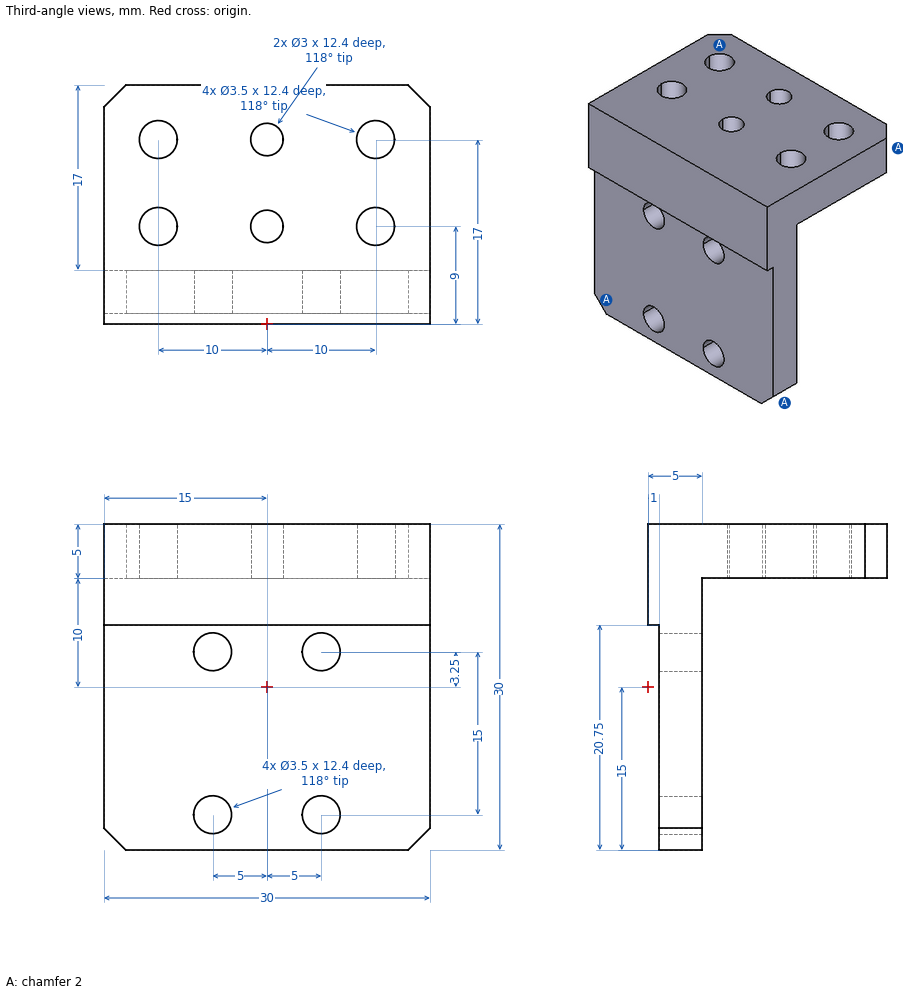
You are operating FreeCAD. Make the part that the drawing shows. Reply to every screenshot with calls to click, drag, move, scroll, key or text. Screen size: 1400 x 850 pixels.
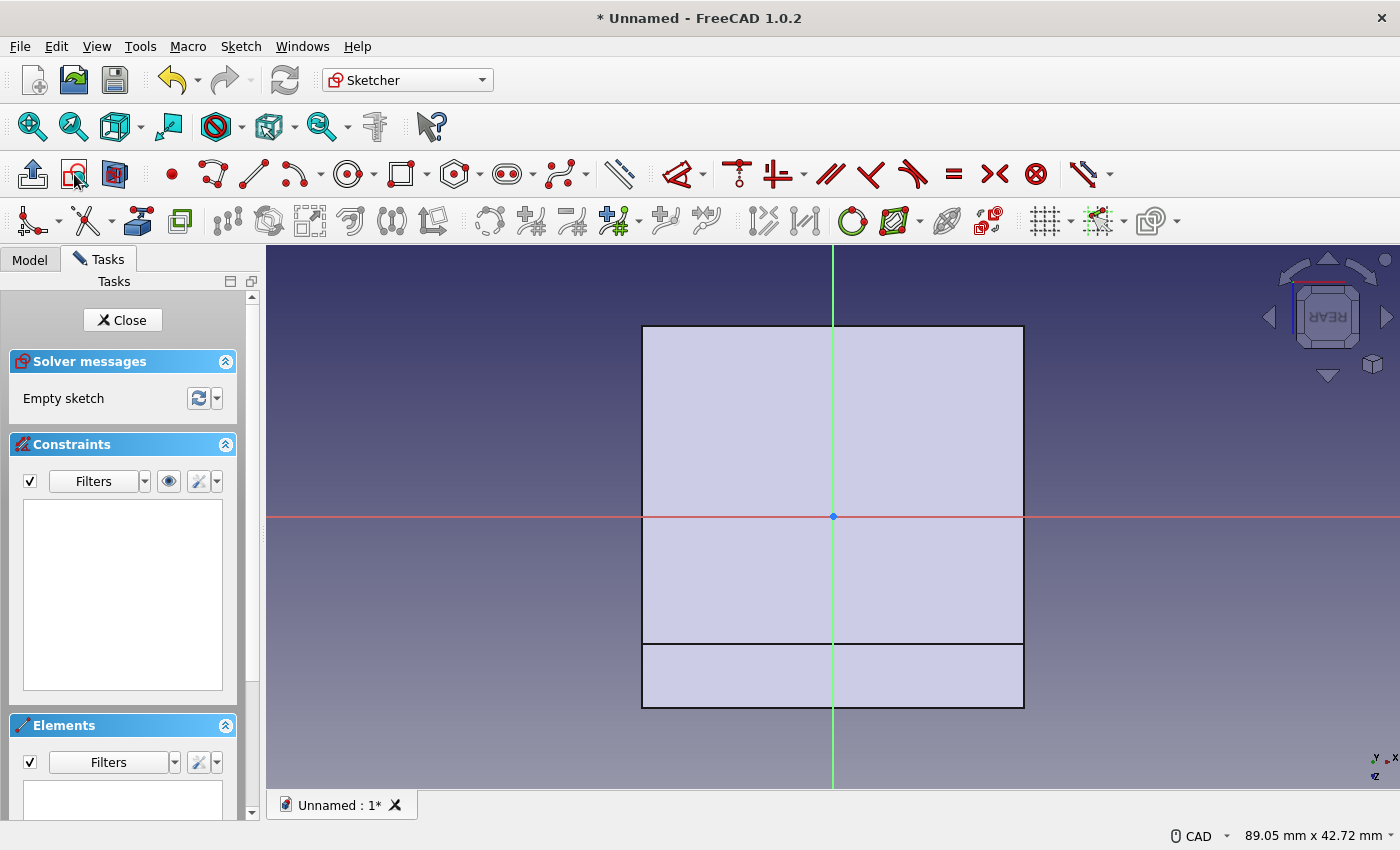
scroll(972, 353, up, 2)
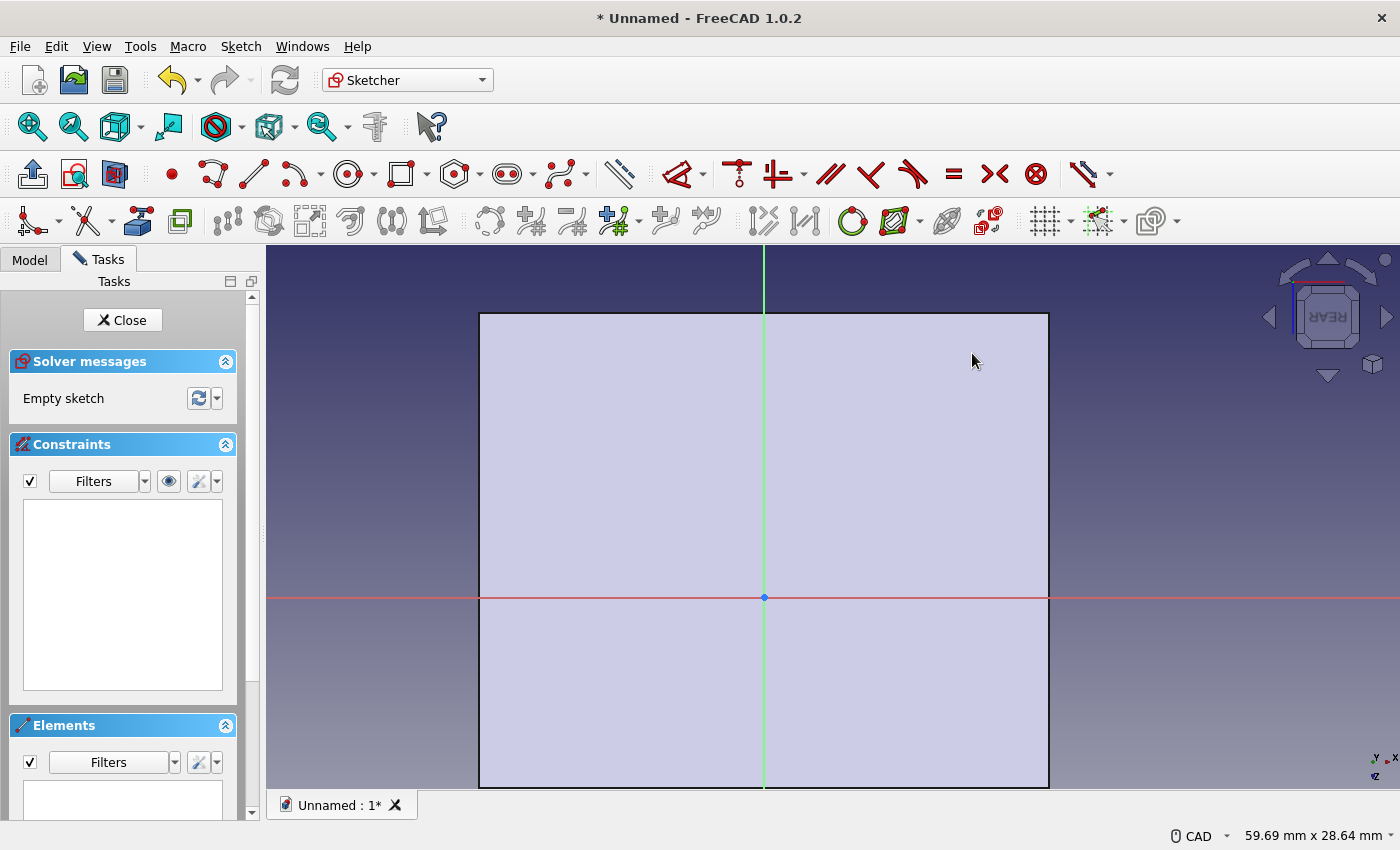
click(348, 174)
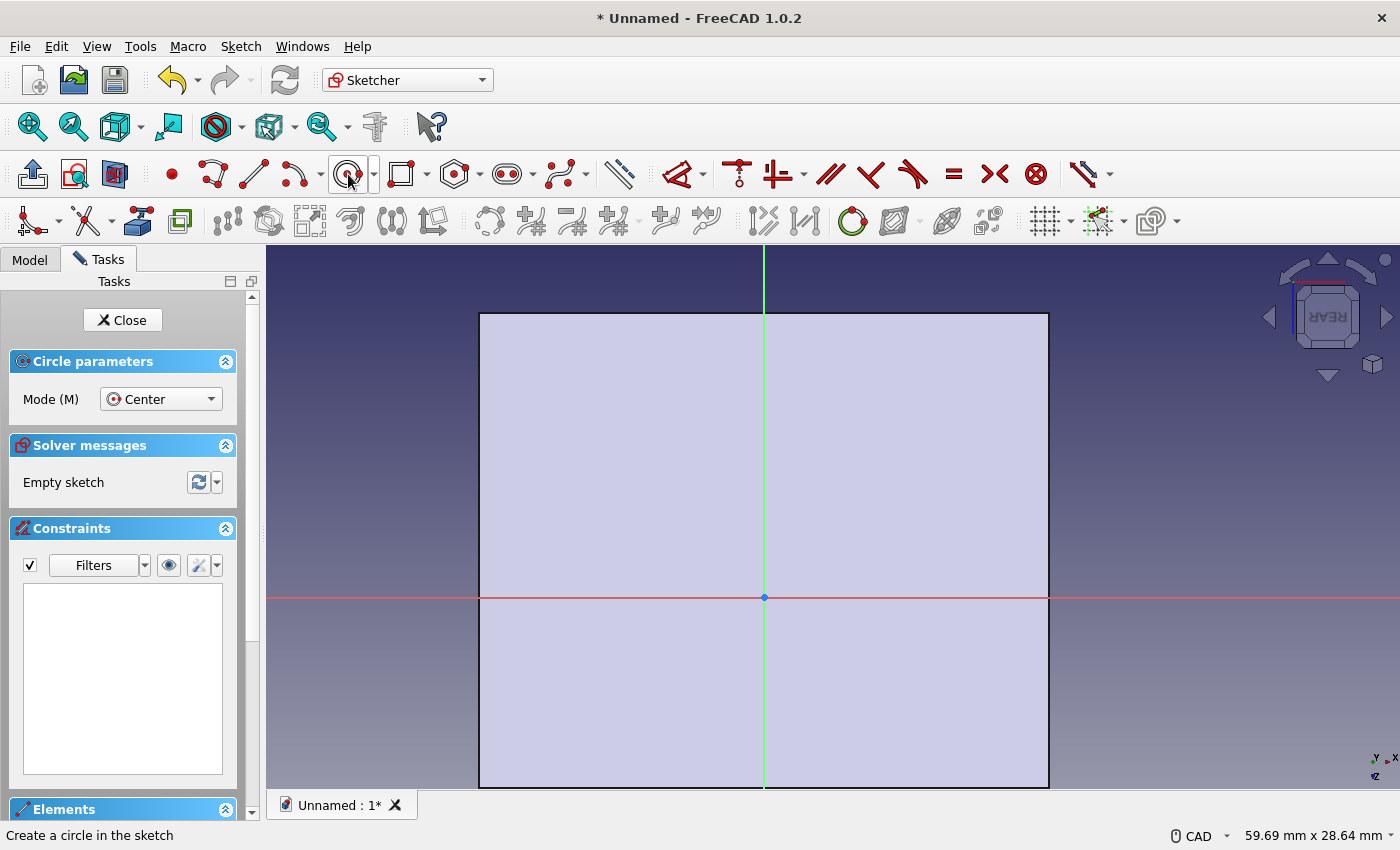
click(669, 374)
click(693, 351)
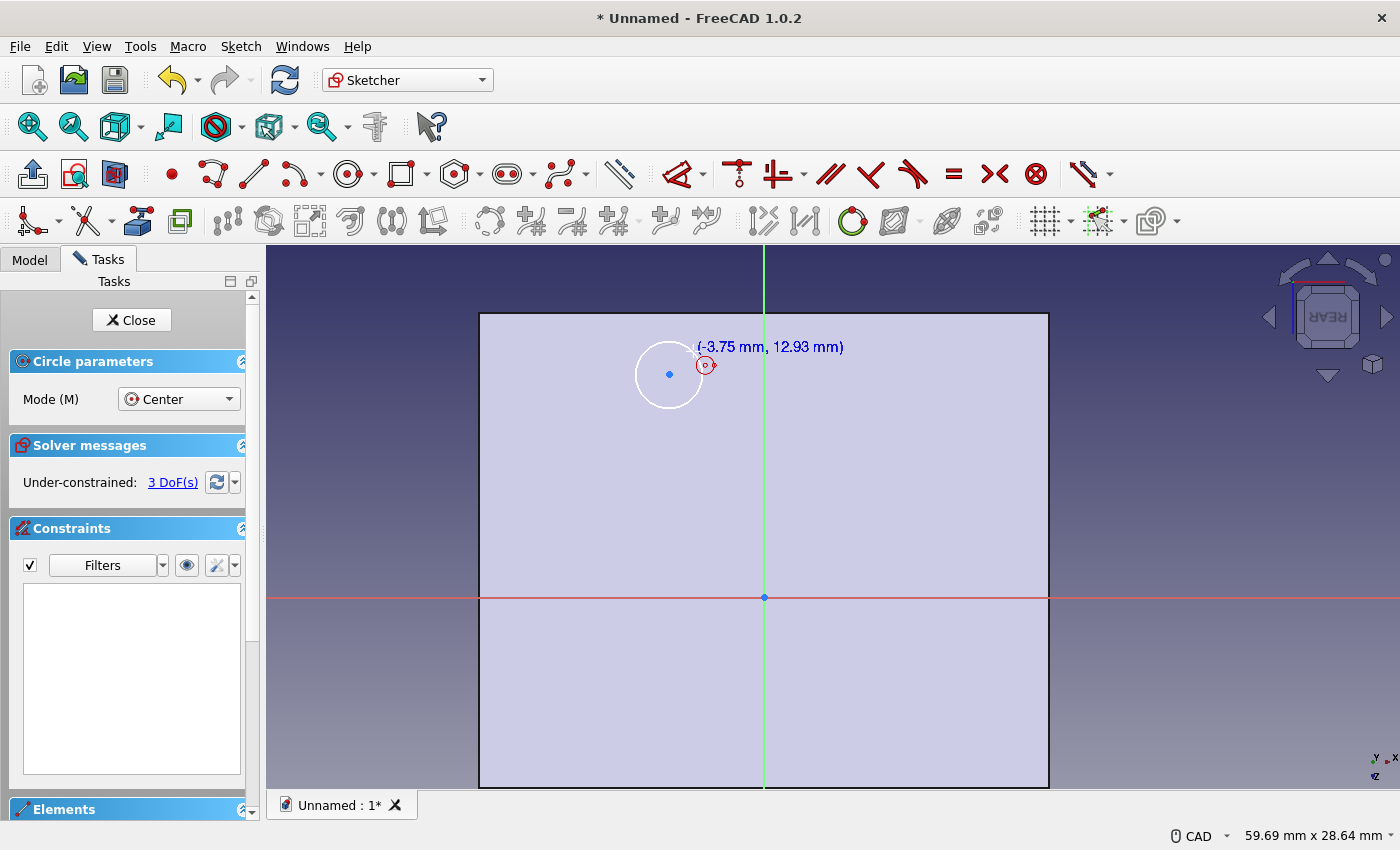
click(859, 374)
click(883, 351)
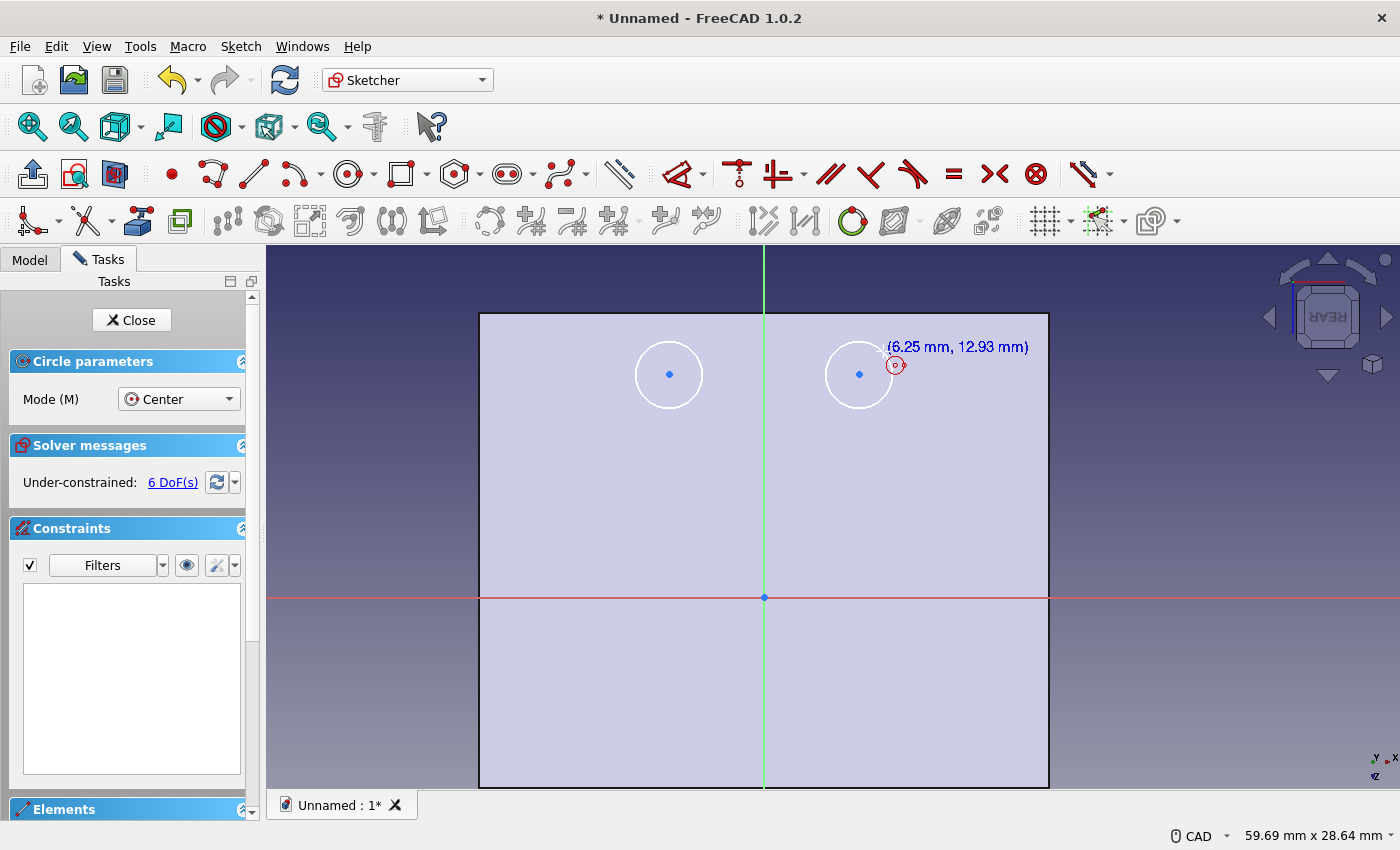
click(859, 659)
click(883, 636)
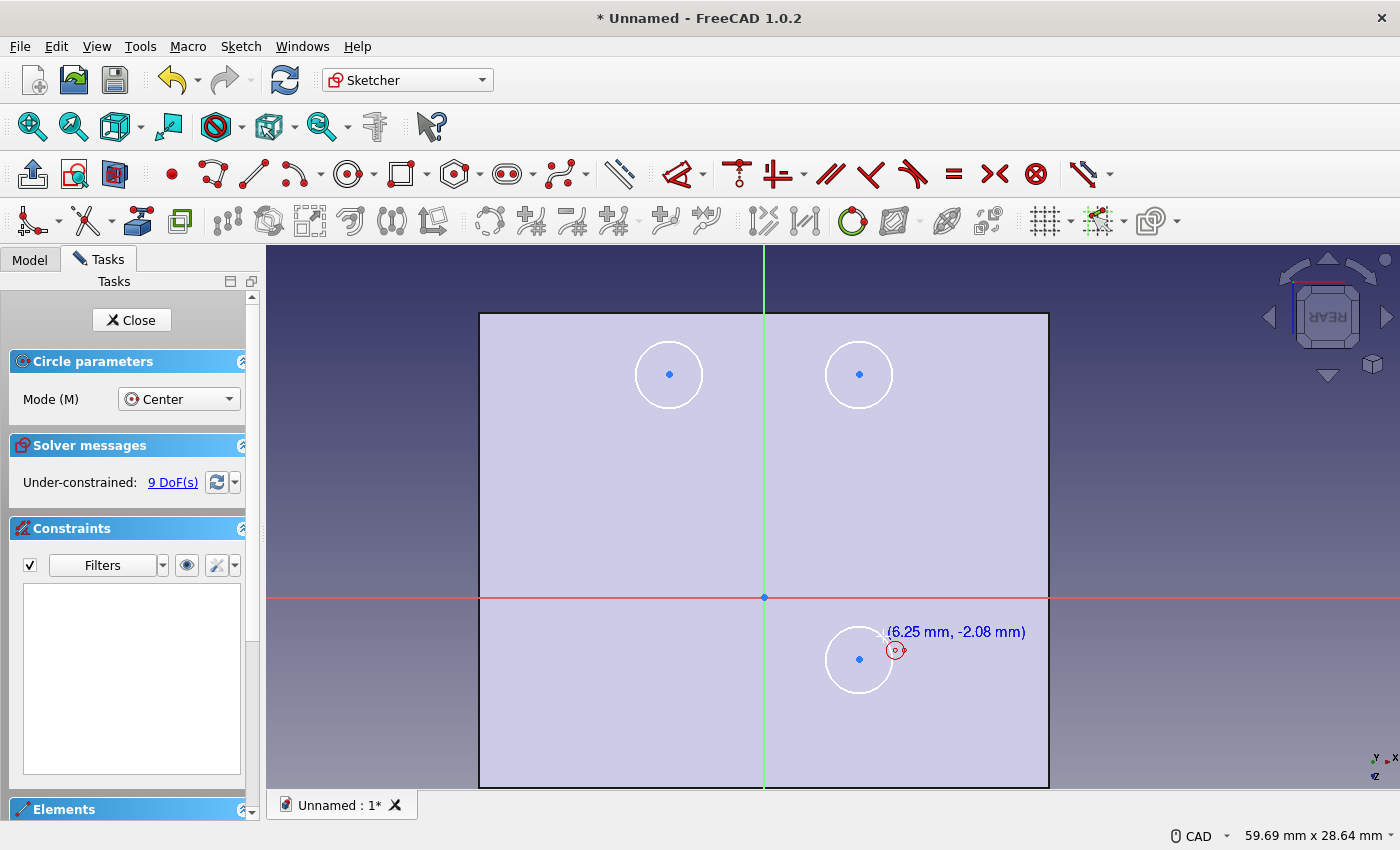
click(669, 659)
click(693, 636)
key(Escape)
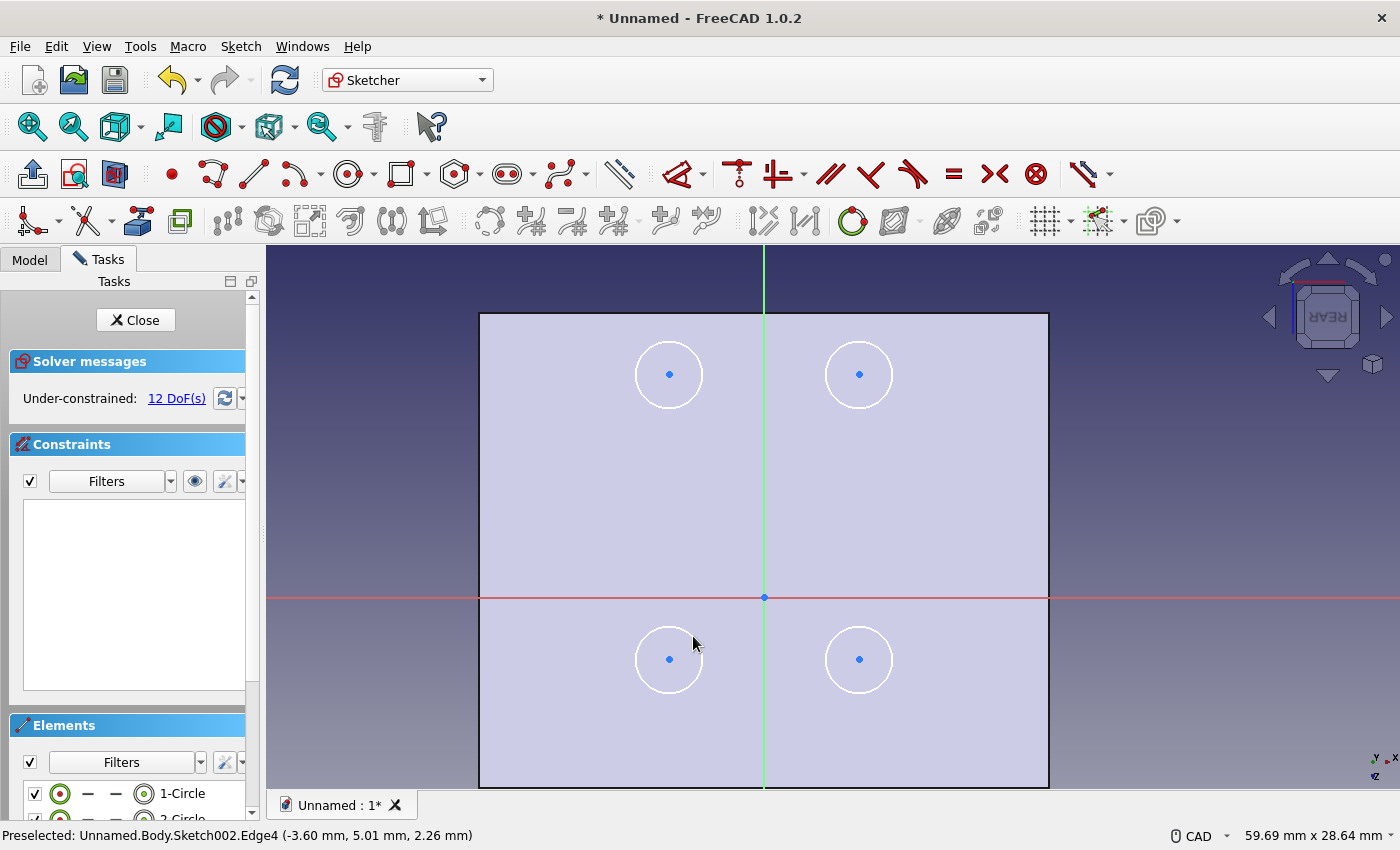
click(692, 351)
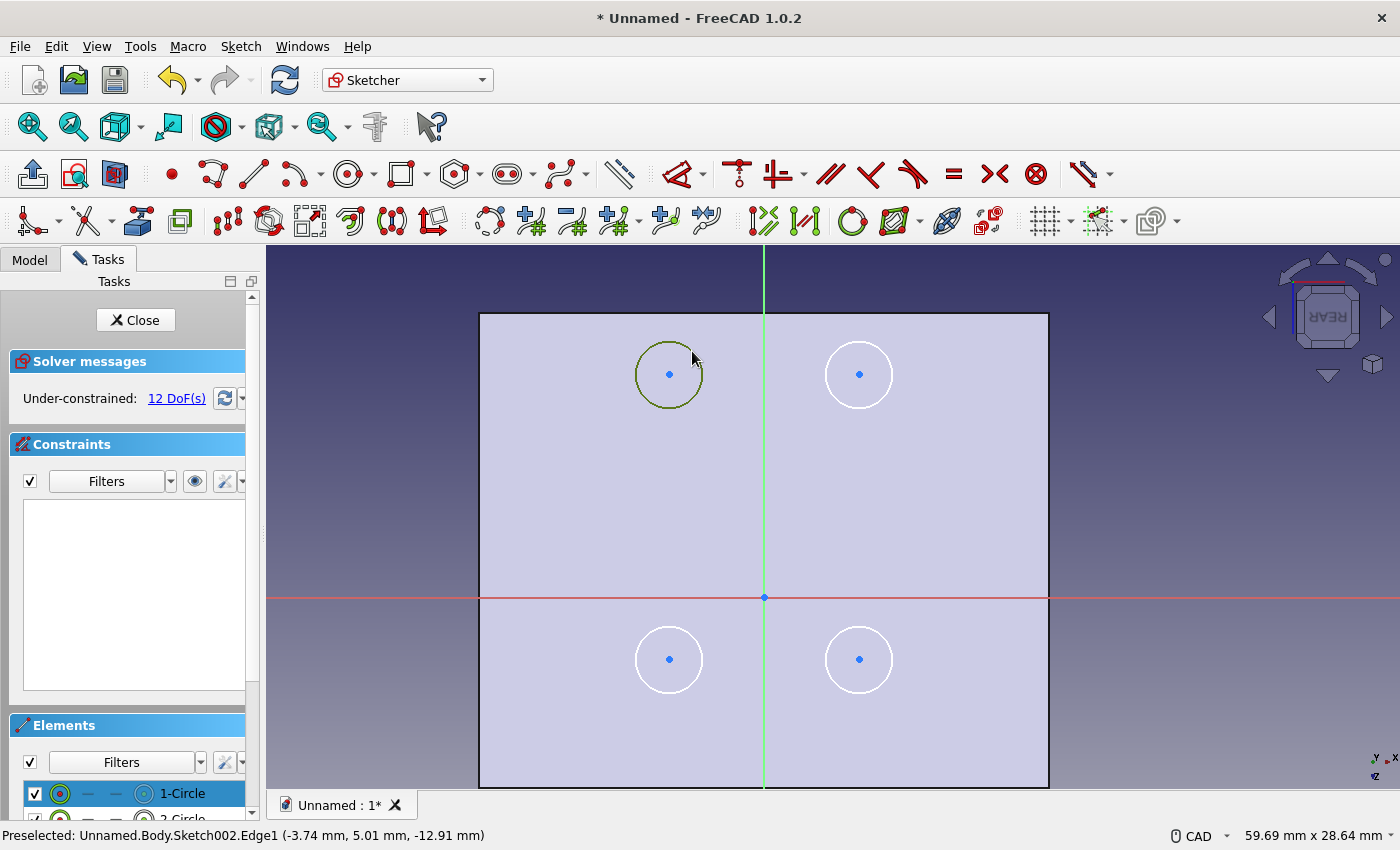
click(882, 351)